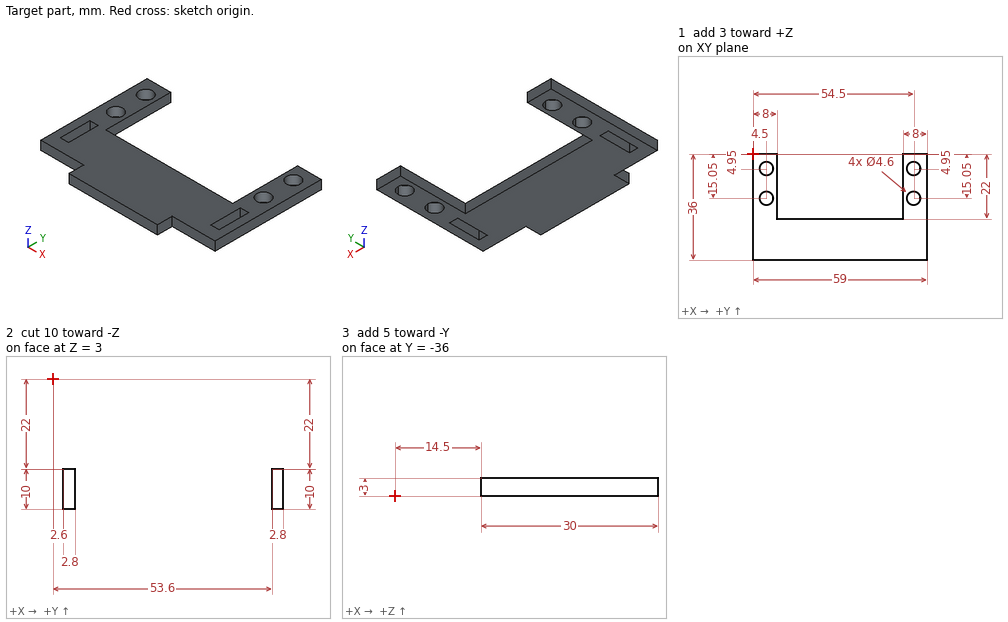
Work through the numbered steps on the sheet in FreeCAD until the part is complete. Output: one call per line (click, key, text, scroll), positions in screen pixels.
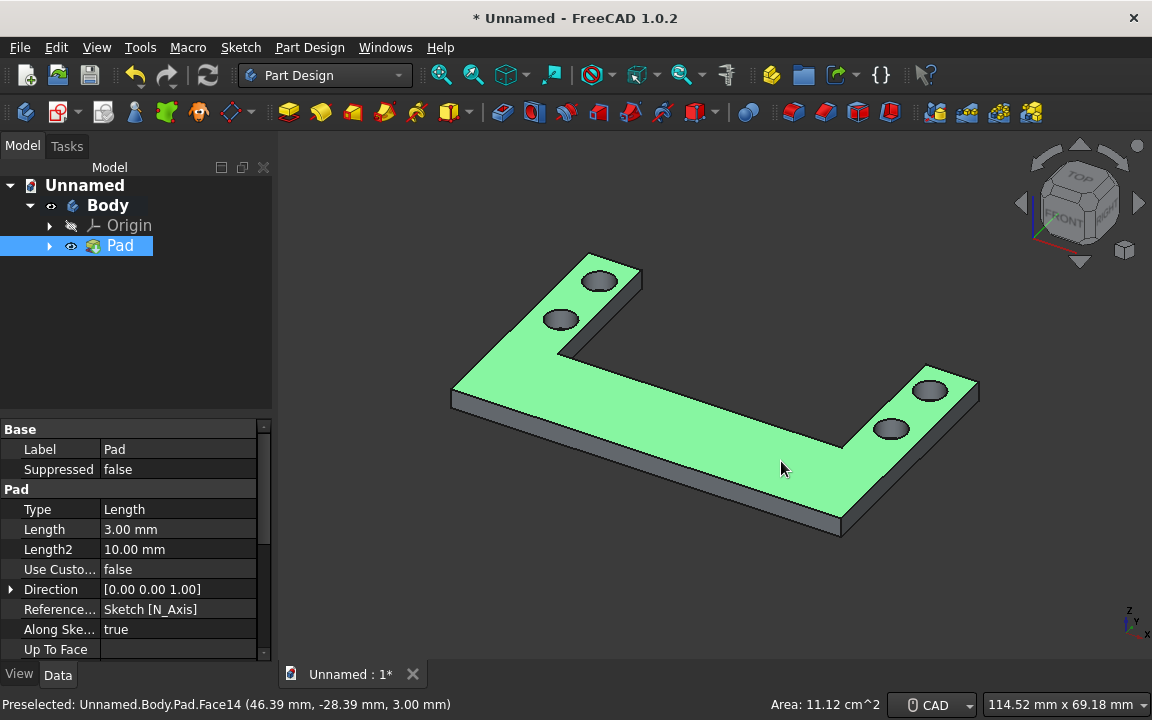
click(58, 112)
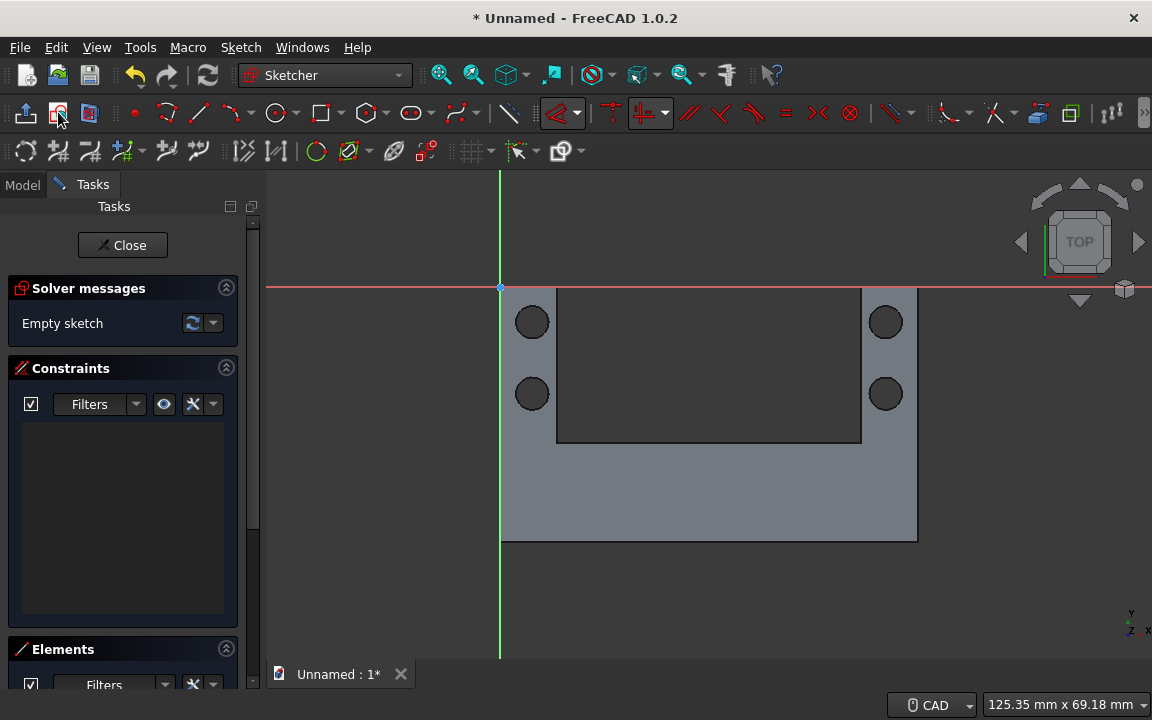
click(322, 114)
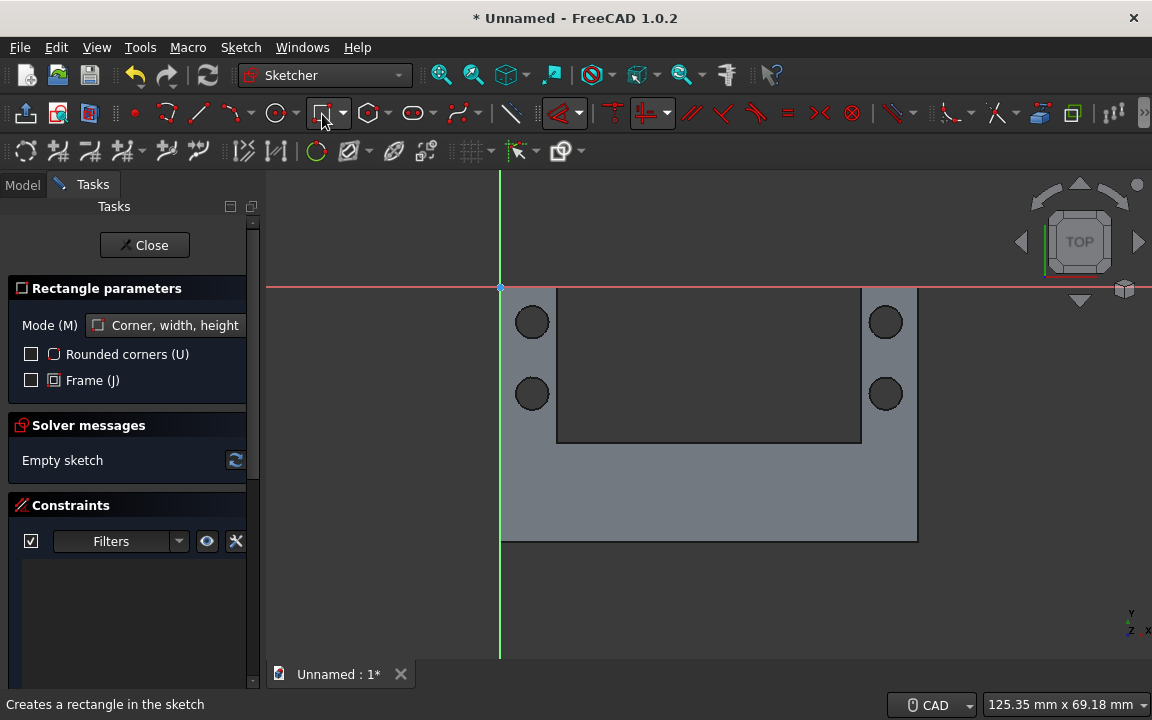
click(519, 443)
click(539, 513)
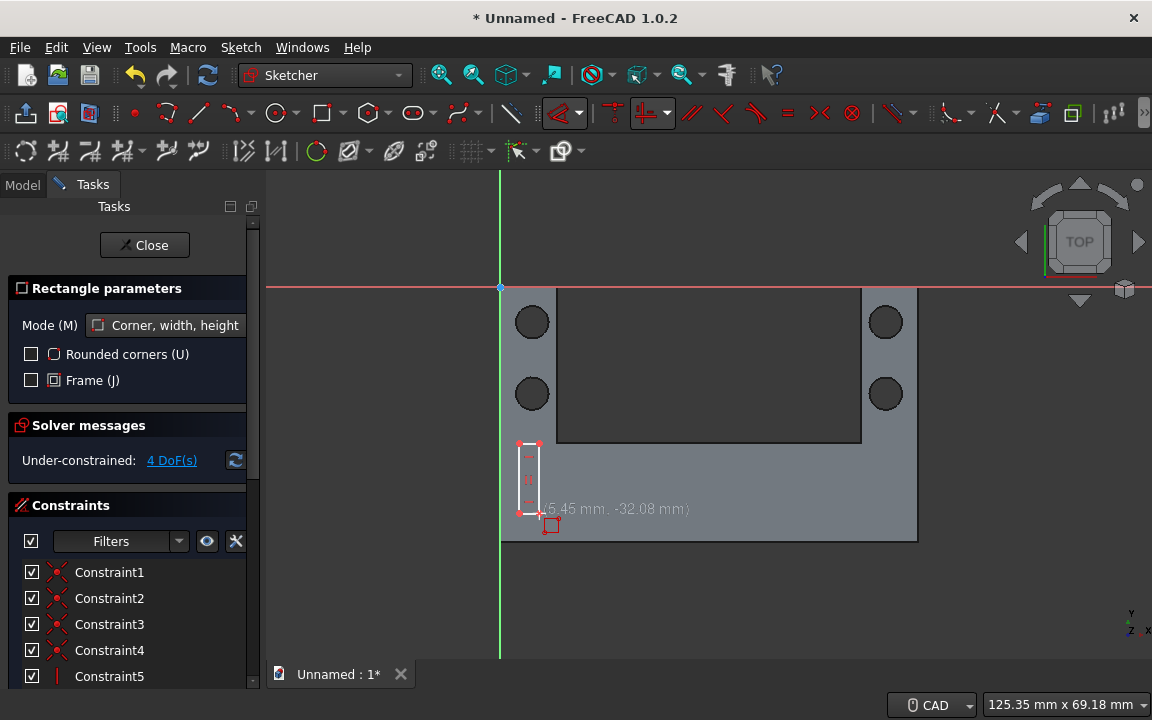
click(879, 443)
click(899, 513)
key(Escape)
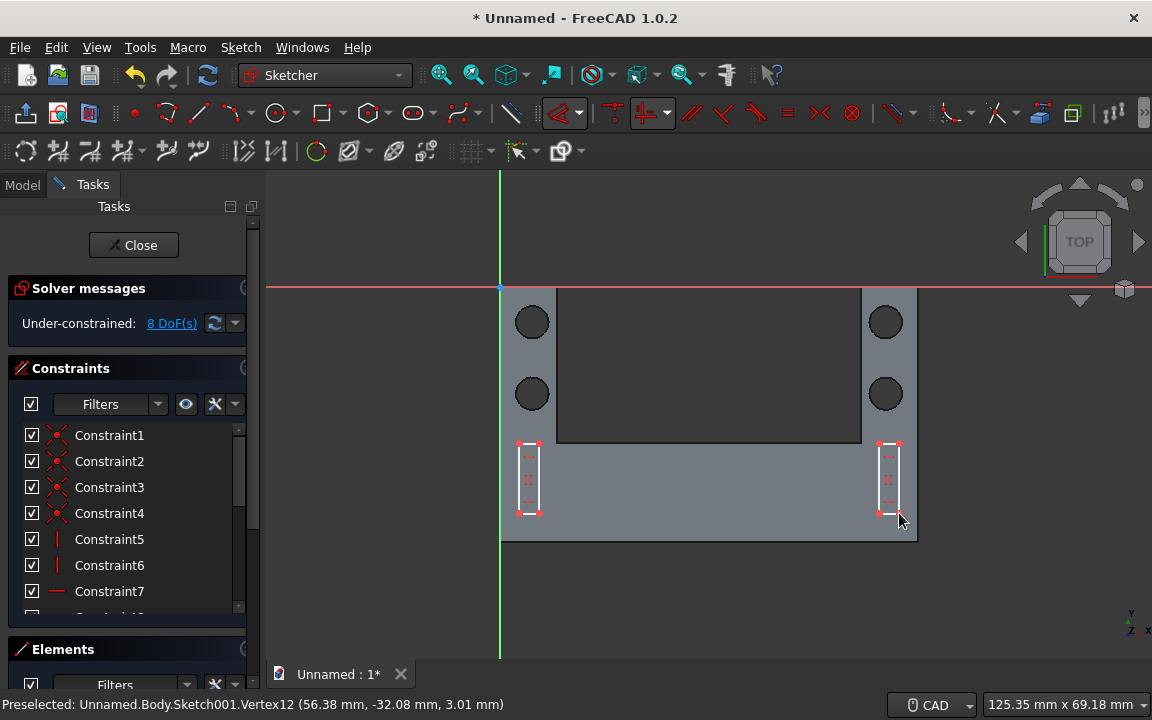
key(d)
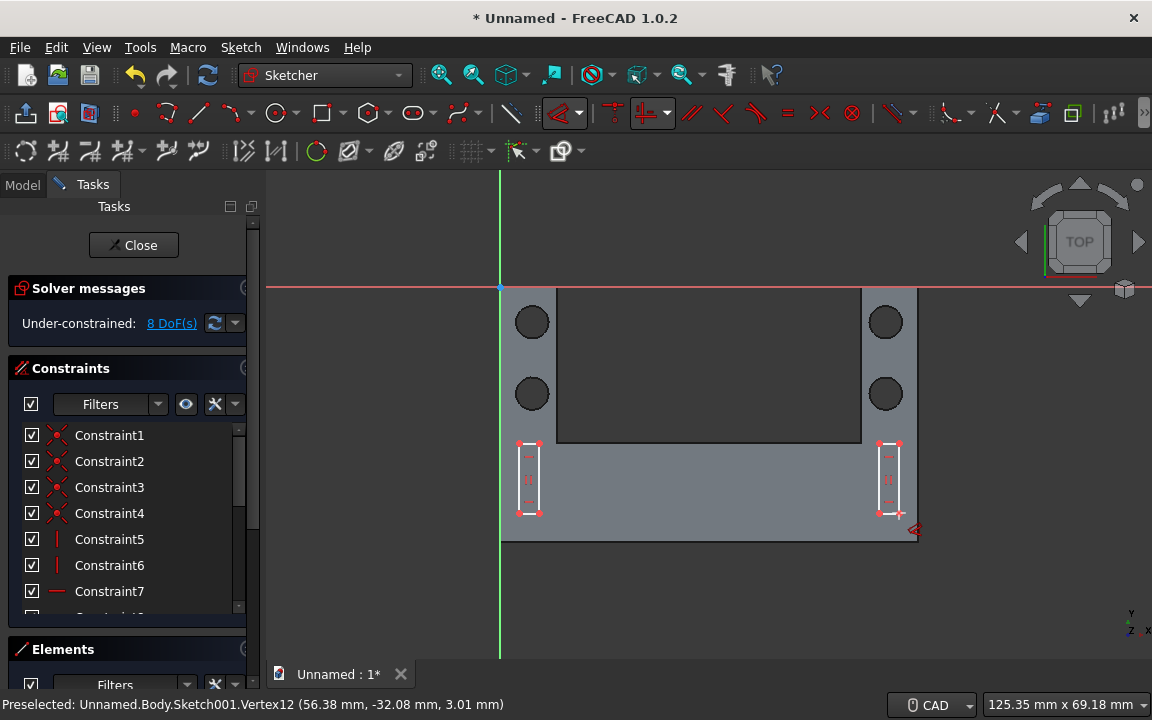
click(519, 465)
click(485, 479)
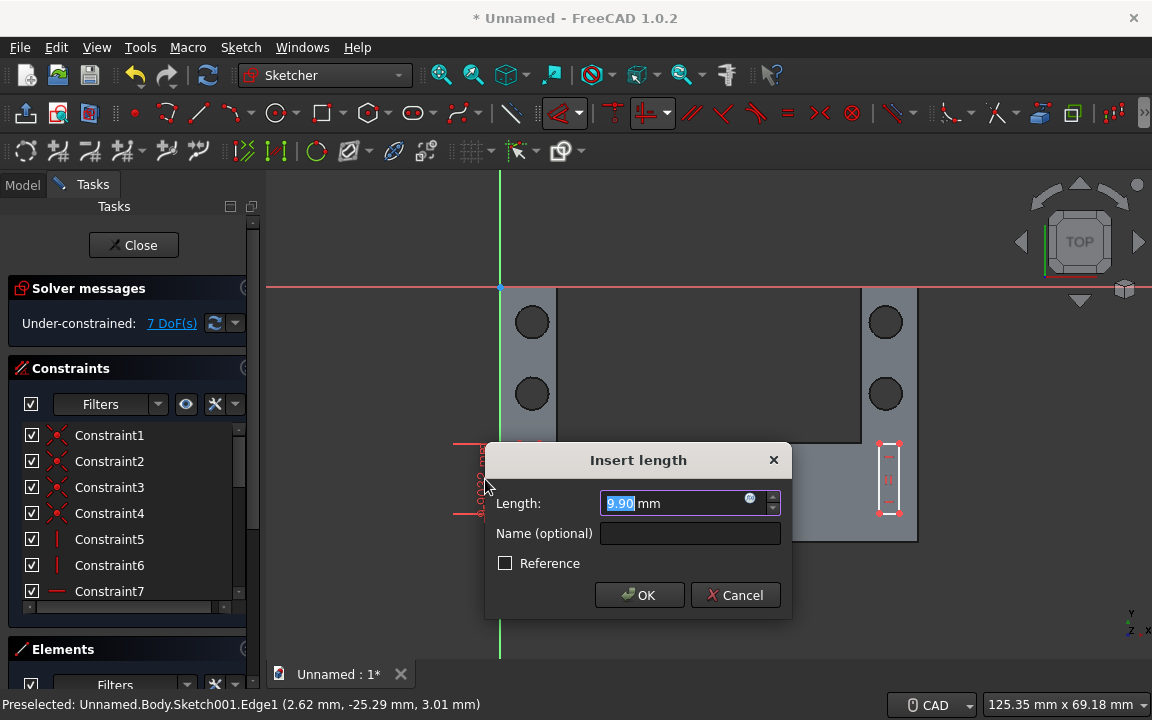
text(10)
key(Return)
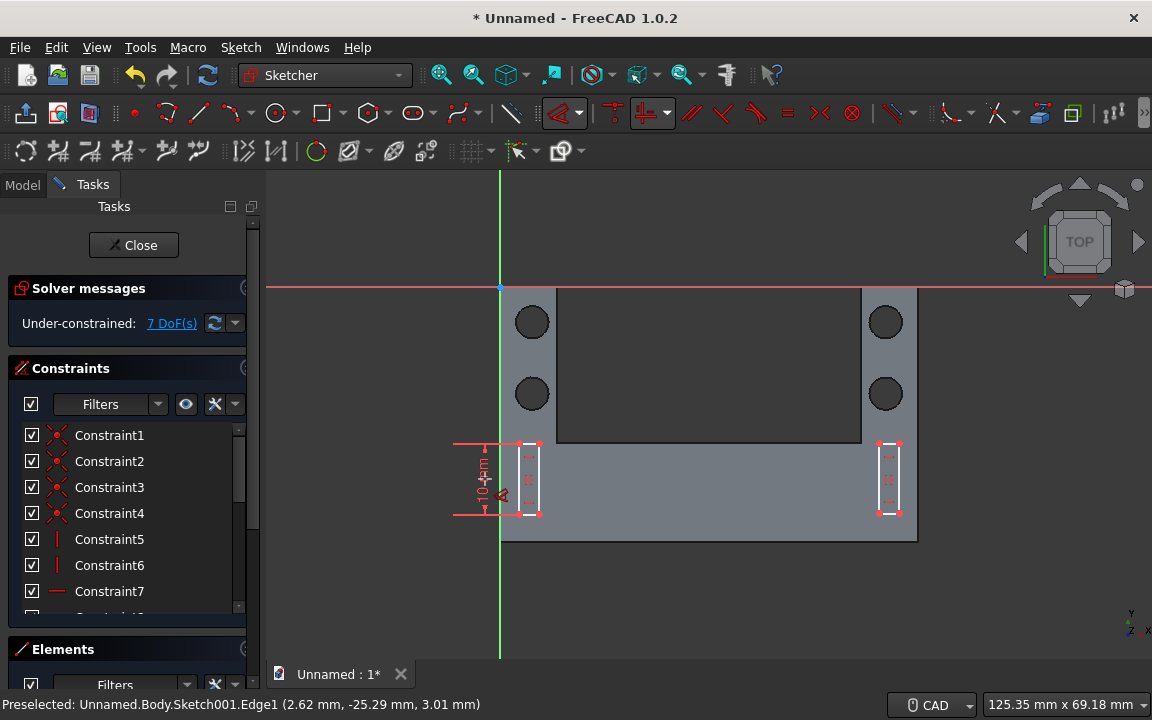
click(879, 465)
click(913, 479)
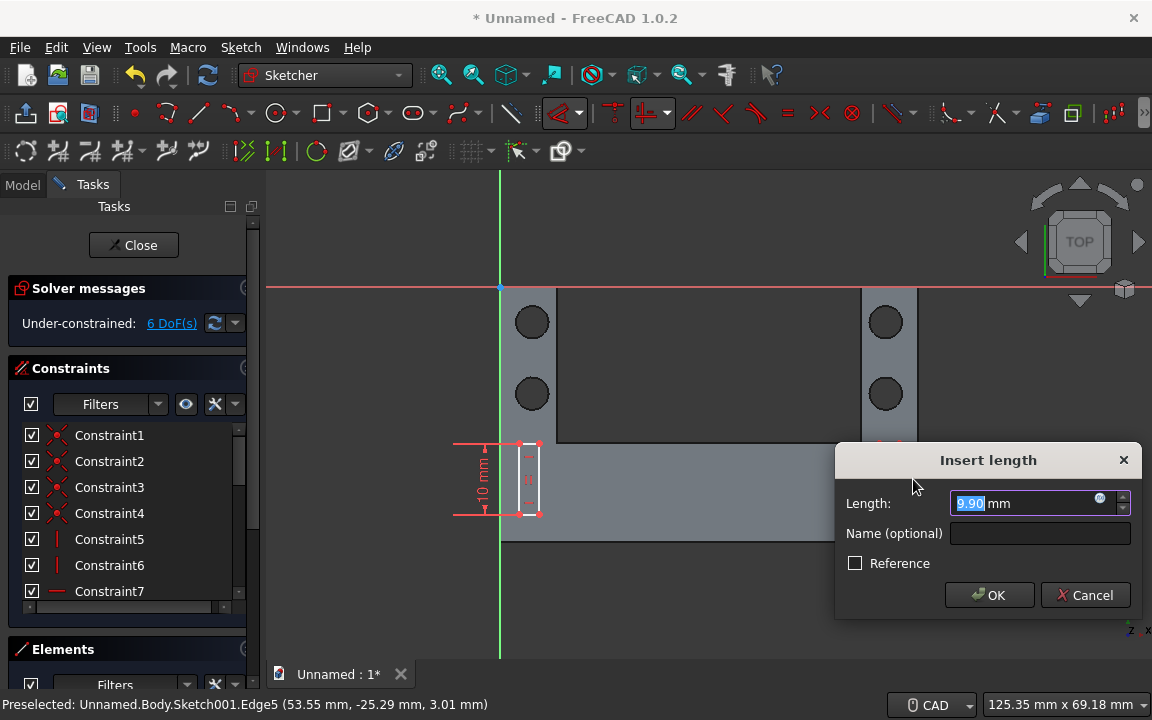
text(10)
key(Return)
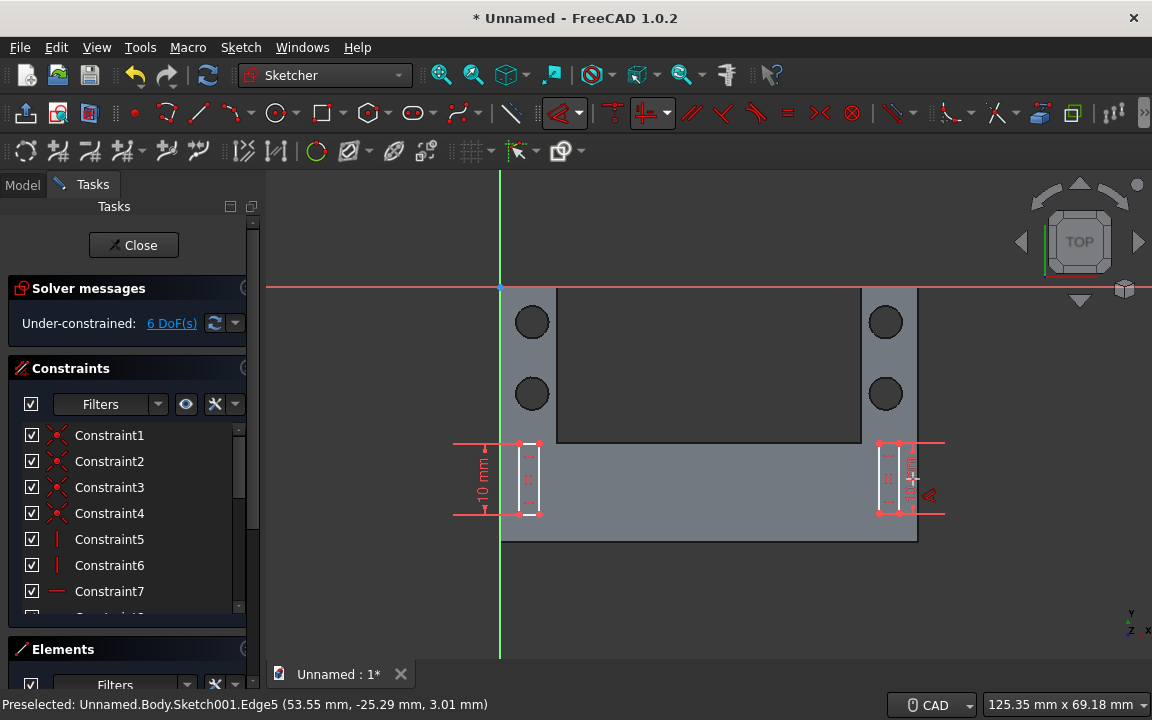
scroll(529, 515, up, 4)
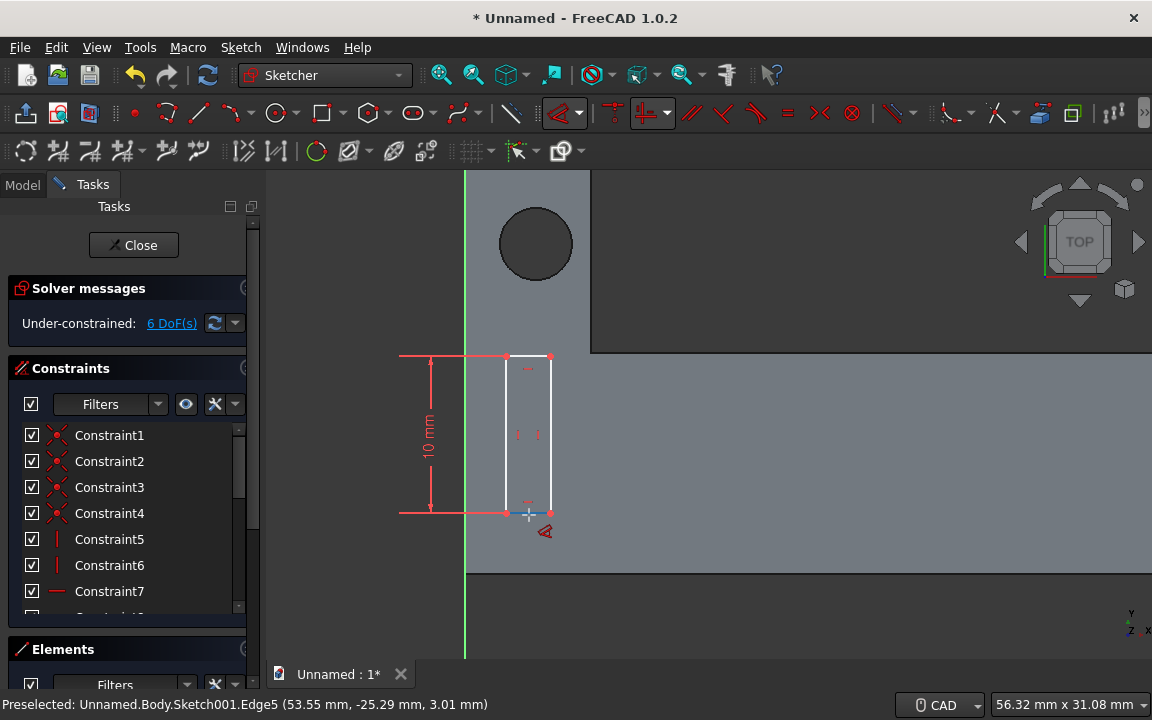
click(529, 513)
click(529, 547)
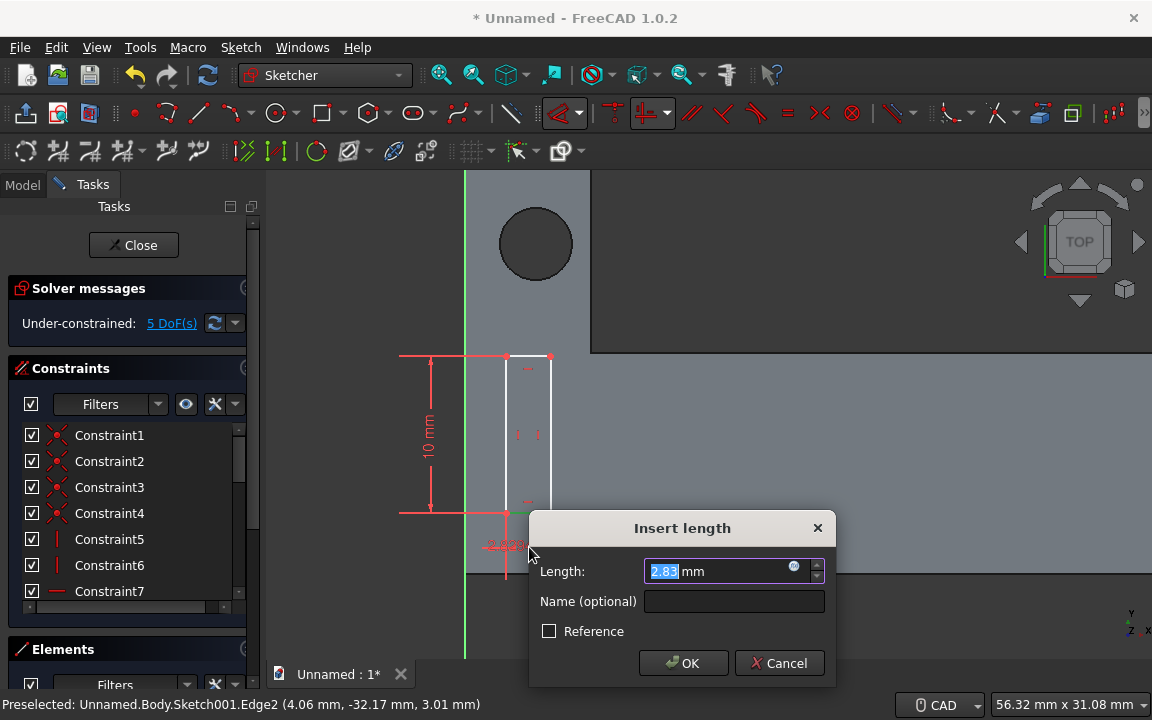
text(2.8)
key(Return)